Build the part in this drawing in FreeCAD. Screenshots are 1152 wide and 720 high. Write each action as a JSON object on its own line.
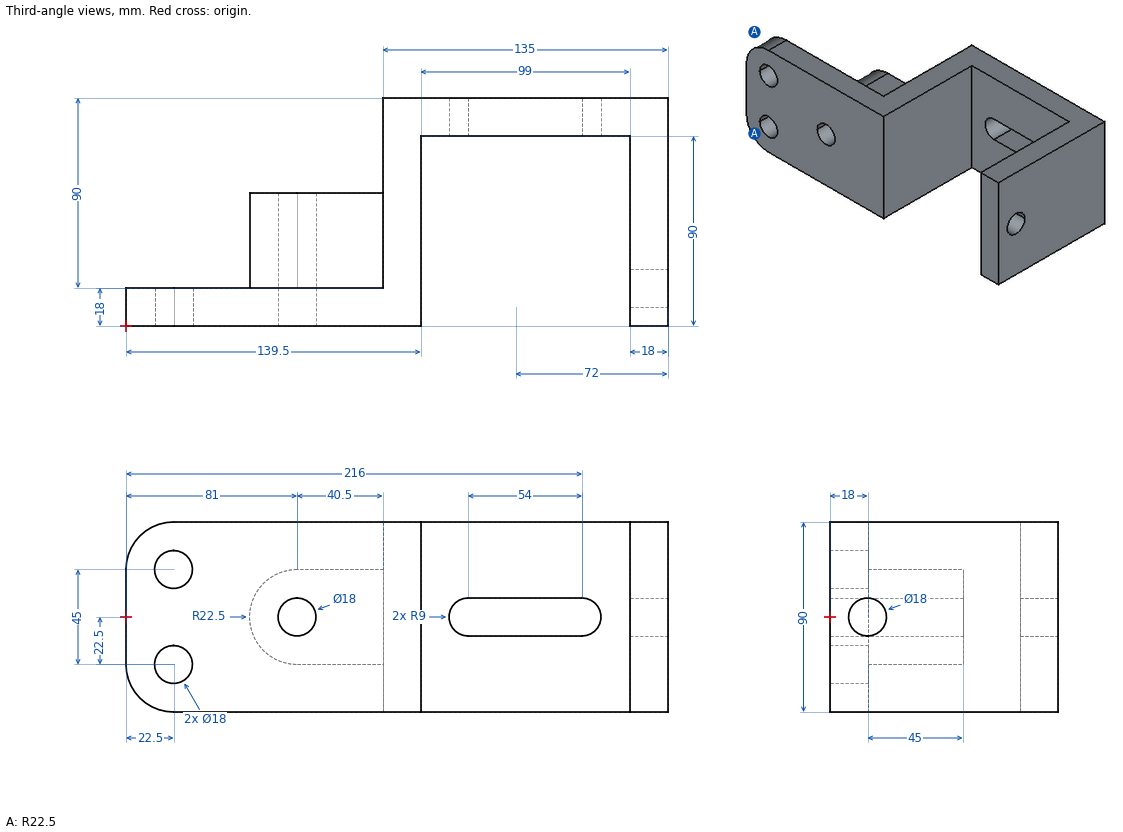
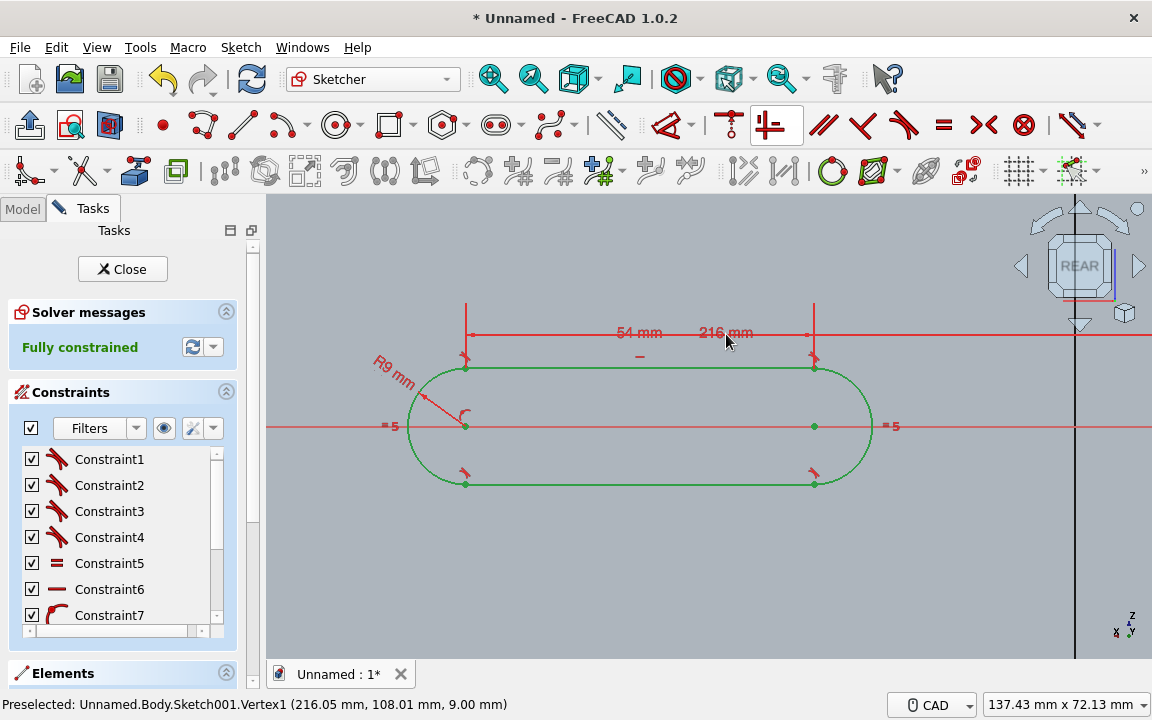
{"action": "left_click", "coordinate": [123, 269]}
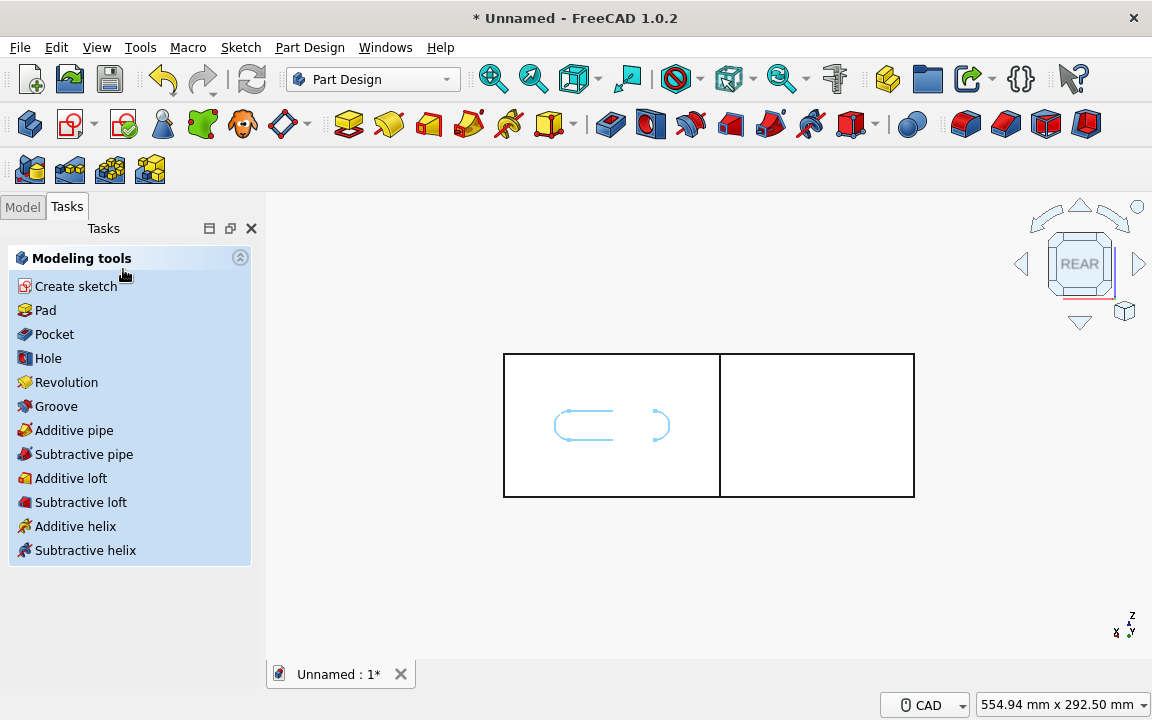
{"action": "left_click", "coordinate": [612, 124]}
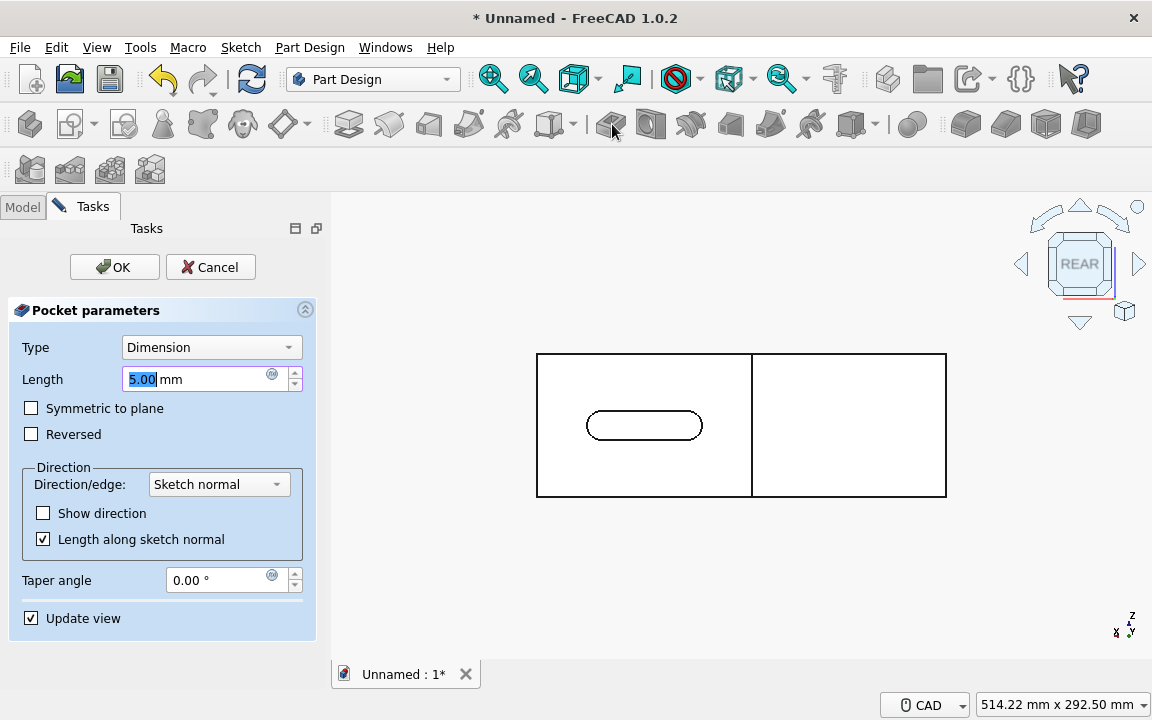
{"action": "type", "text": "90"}
{"action": "key", "text": "Tab"}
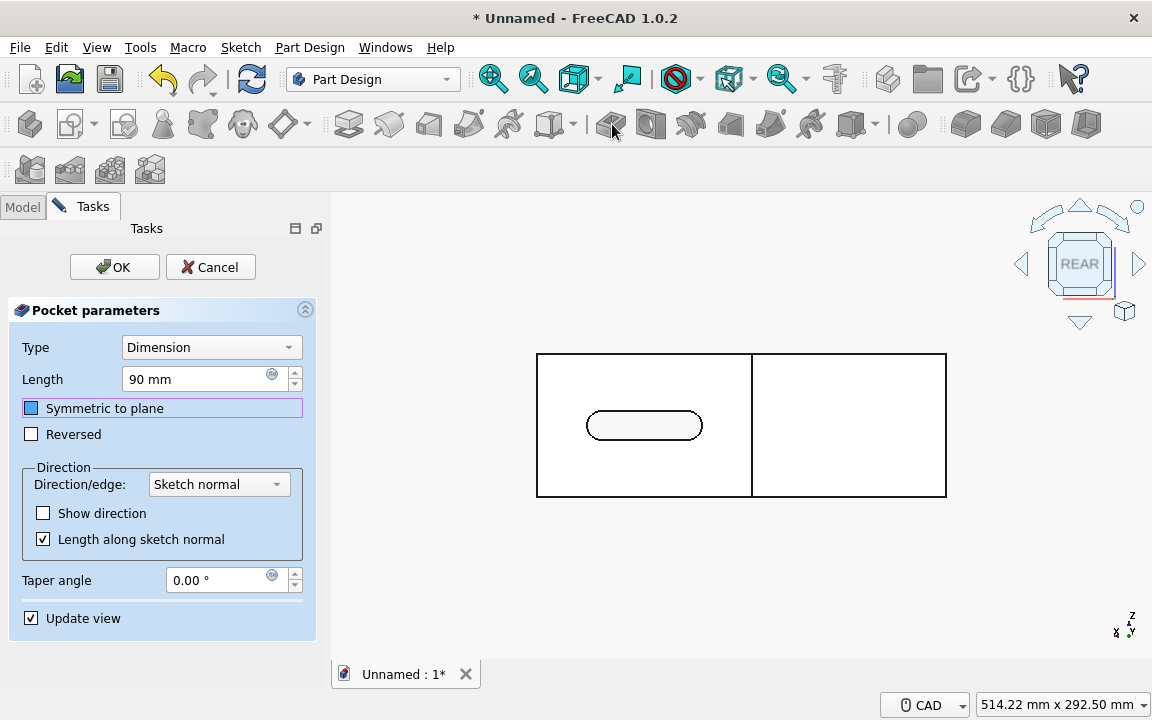
{"action": "left_click", "coordinate": [30, 408]}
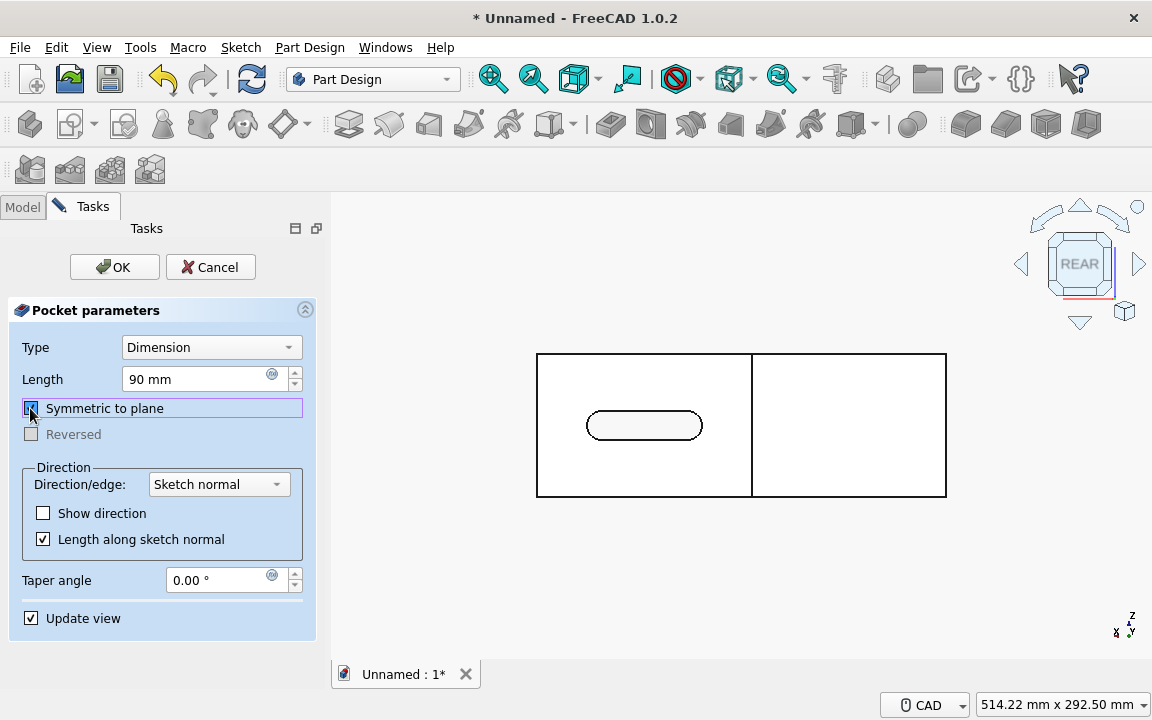
{"action": "left_click", "coordinate": [115, 267]}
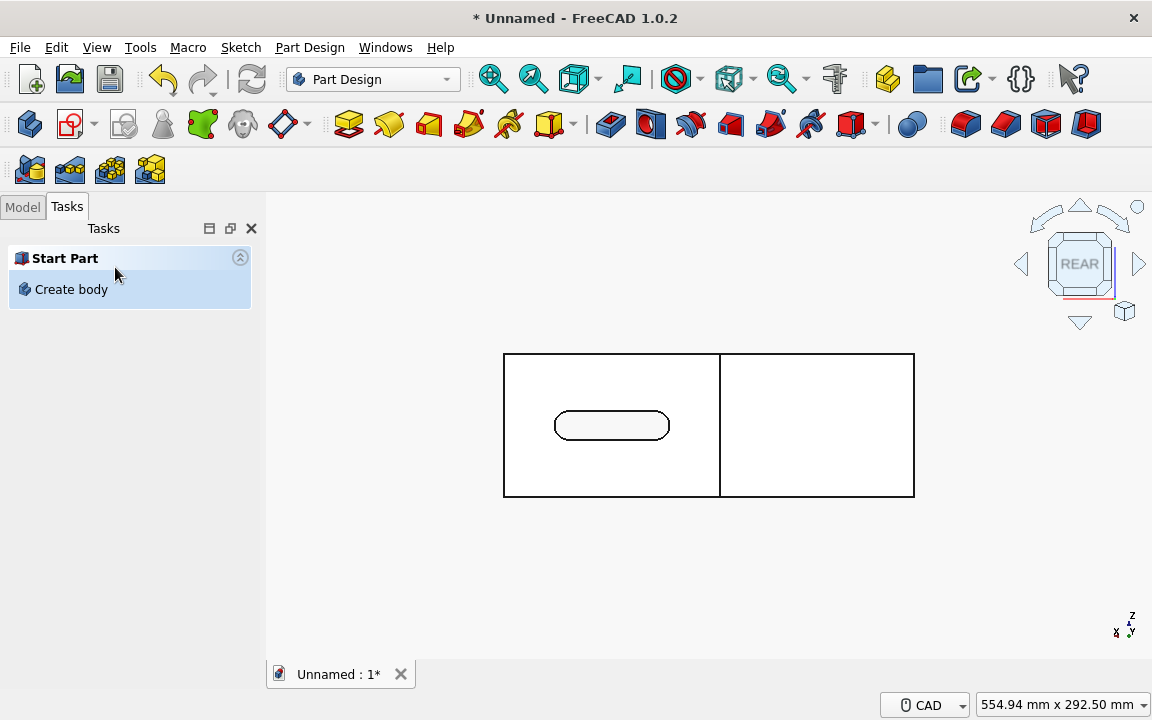
{"action": "left_click", "coordinate": [817, 424]}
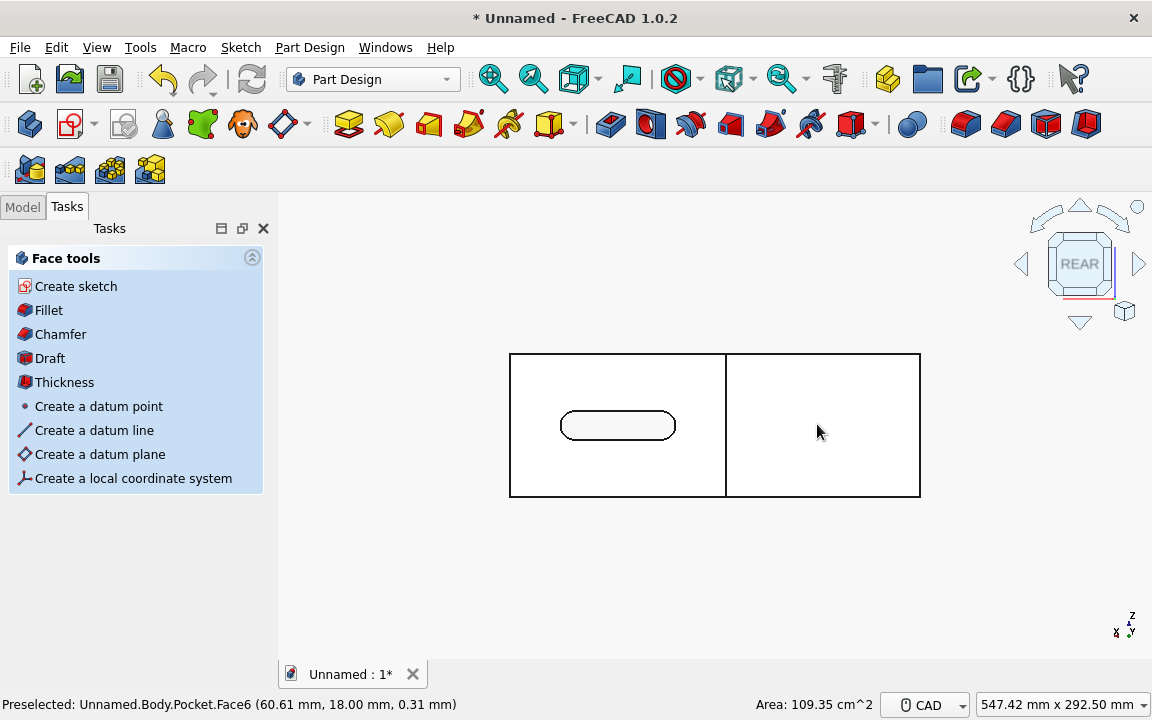
{"action": "left_click", "coordinate": [70, 124]}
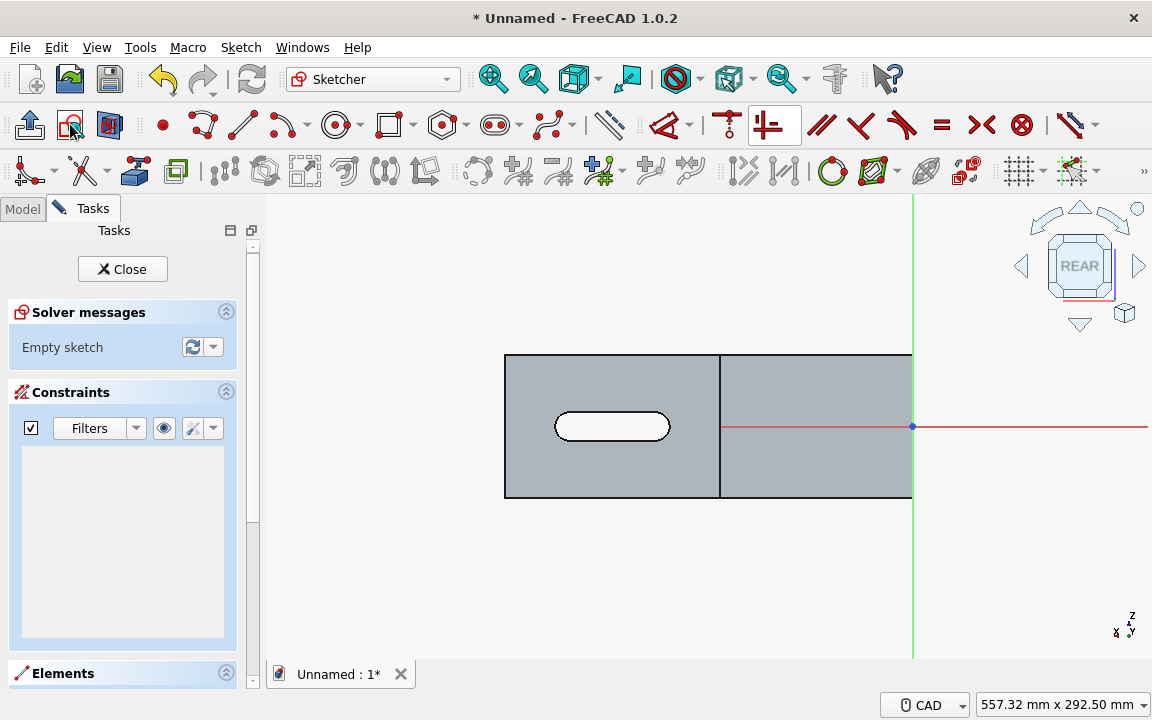
{"action": "left_click", "coordinate": [110, 126]}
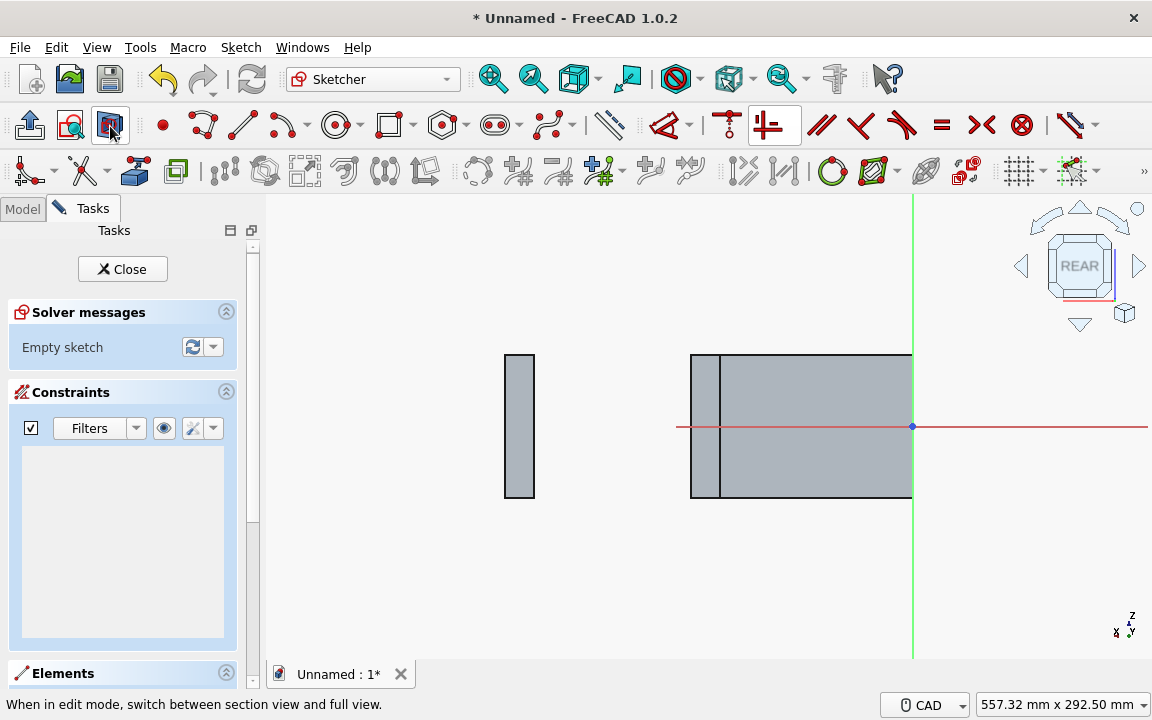
{"action": "scroll", "coordinate": [919, 427], "scroll_direction": "up", "scroll_amount": 5}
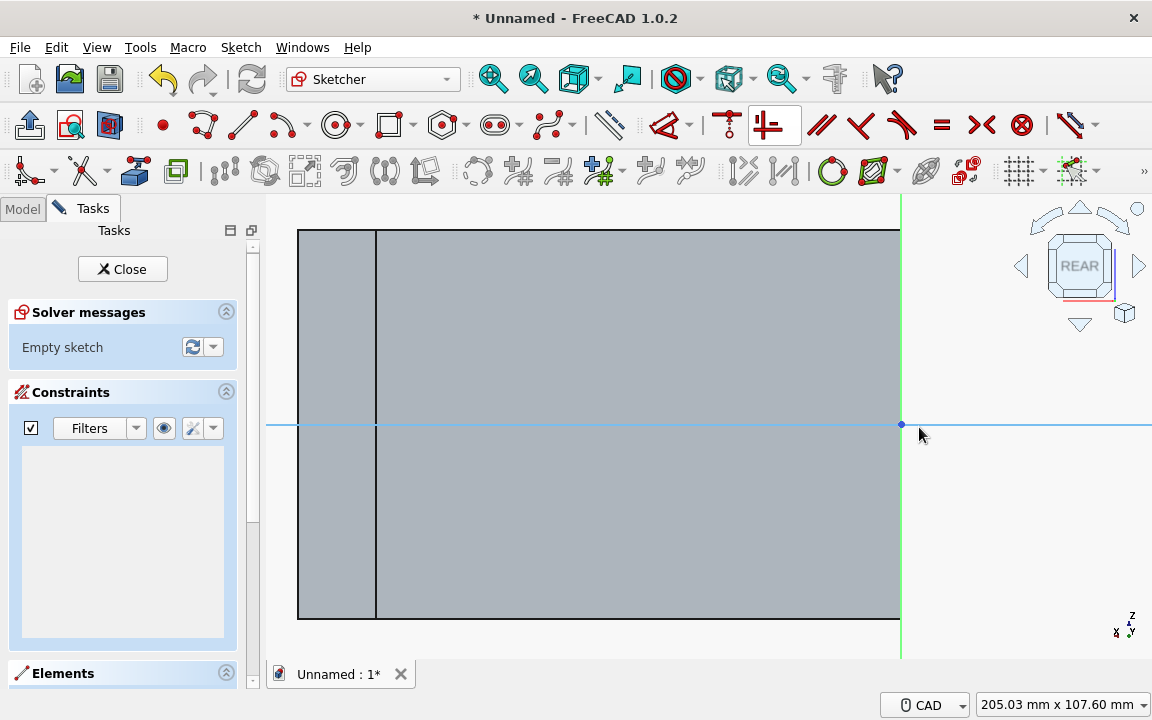
{"action": "key", "text": "g m"}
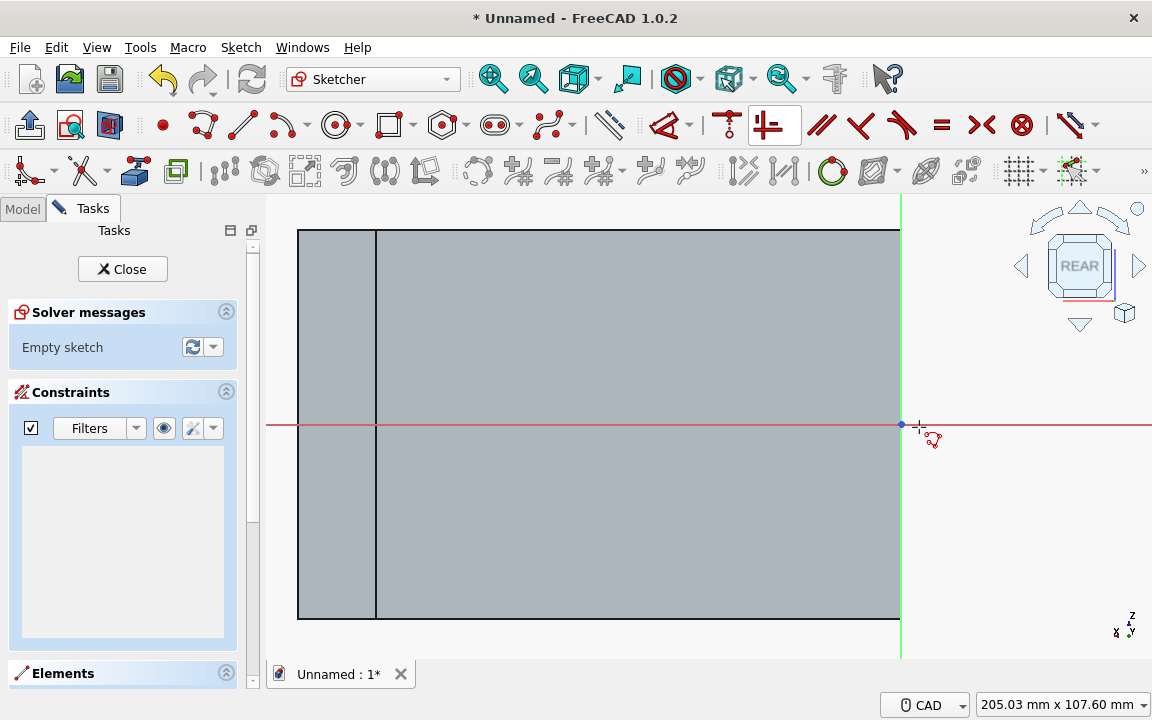
{"action": "left_click", "coordinate": [551, 328]}
{"action": "left_click", "coordinate": [376, 328]}
{"action": "left_click", "coordinate": [376, 522]}
{"action": "left_click", "coordinate": [551, 522]}
{"action": "right_click", "coordinate": [551, 522]}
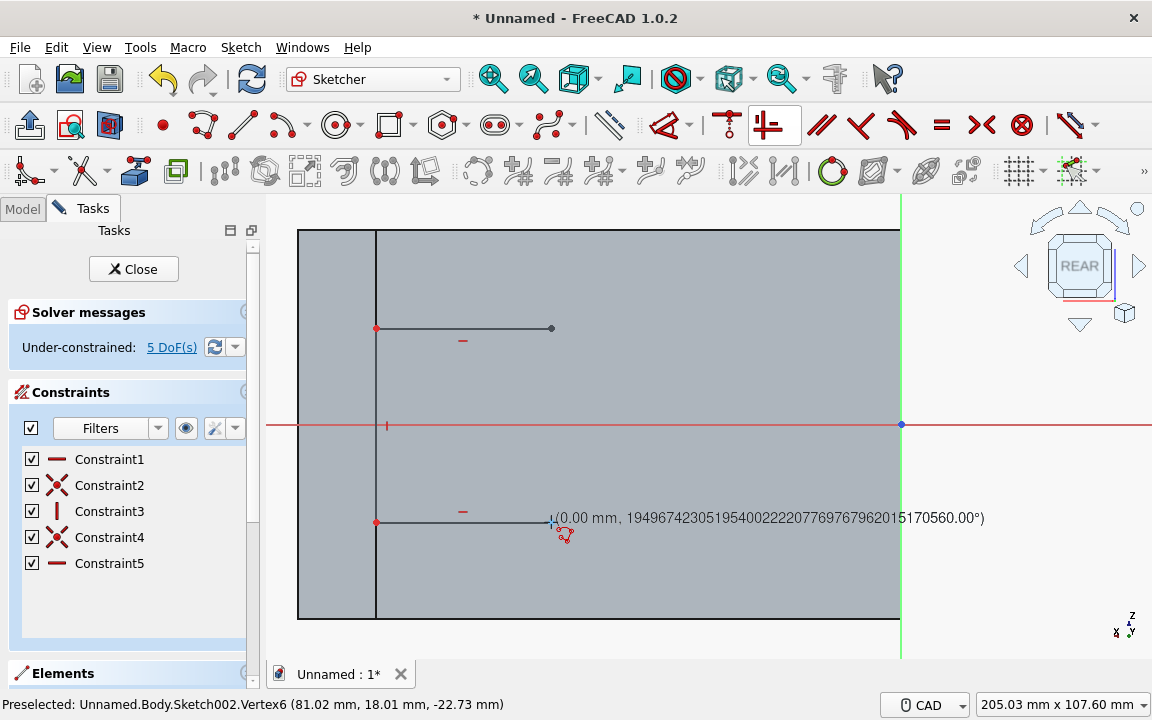
{"action": "key", "text": "g 3 a"}